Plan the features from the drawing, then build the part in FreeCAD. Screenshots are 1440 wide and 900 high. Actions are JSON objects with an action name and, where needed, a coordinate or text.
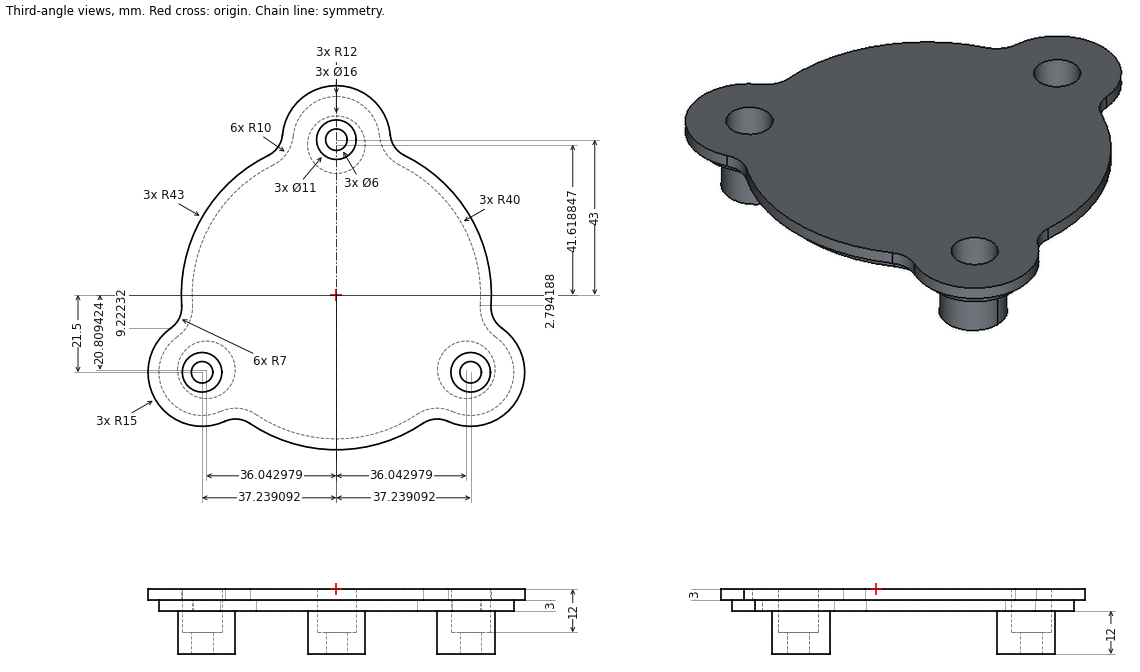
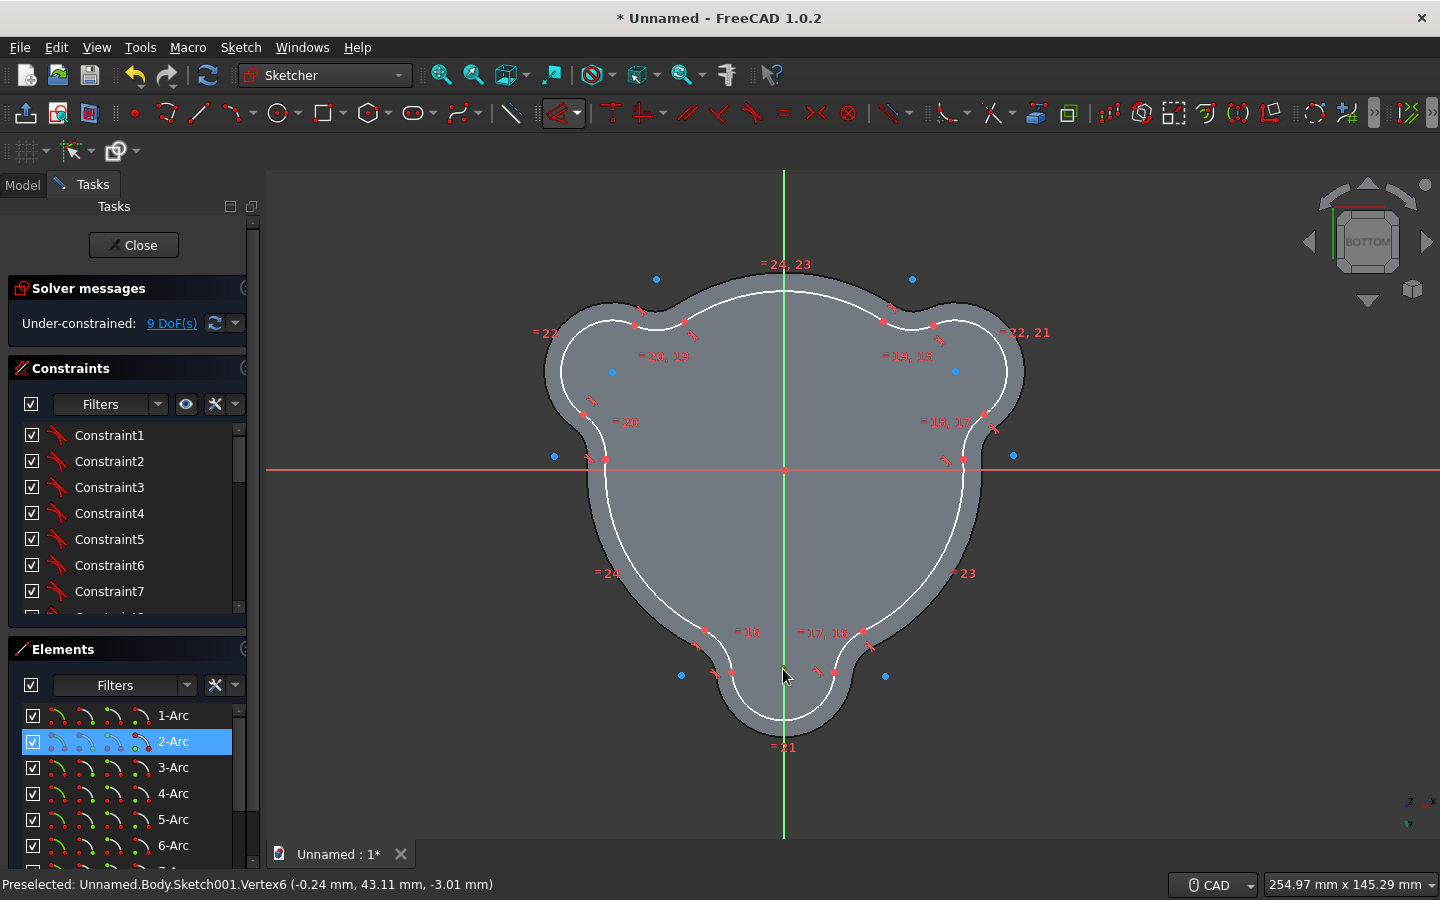
{"action": "left_click", "coordinate": [784, 767]}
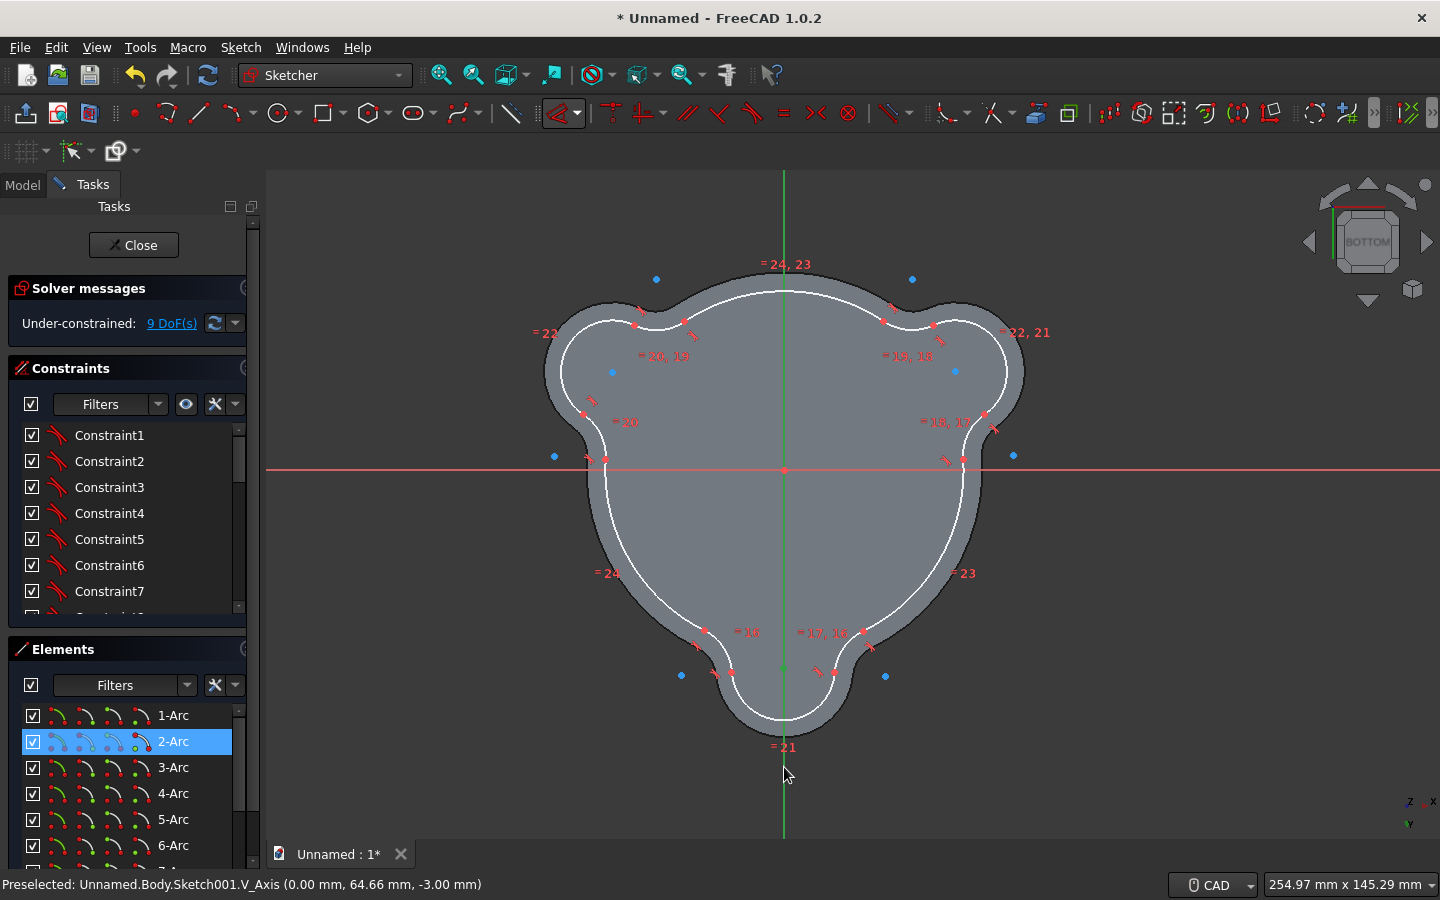
{"action": "left_click", "coordinate": [612, 114]}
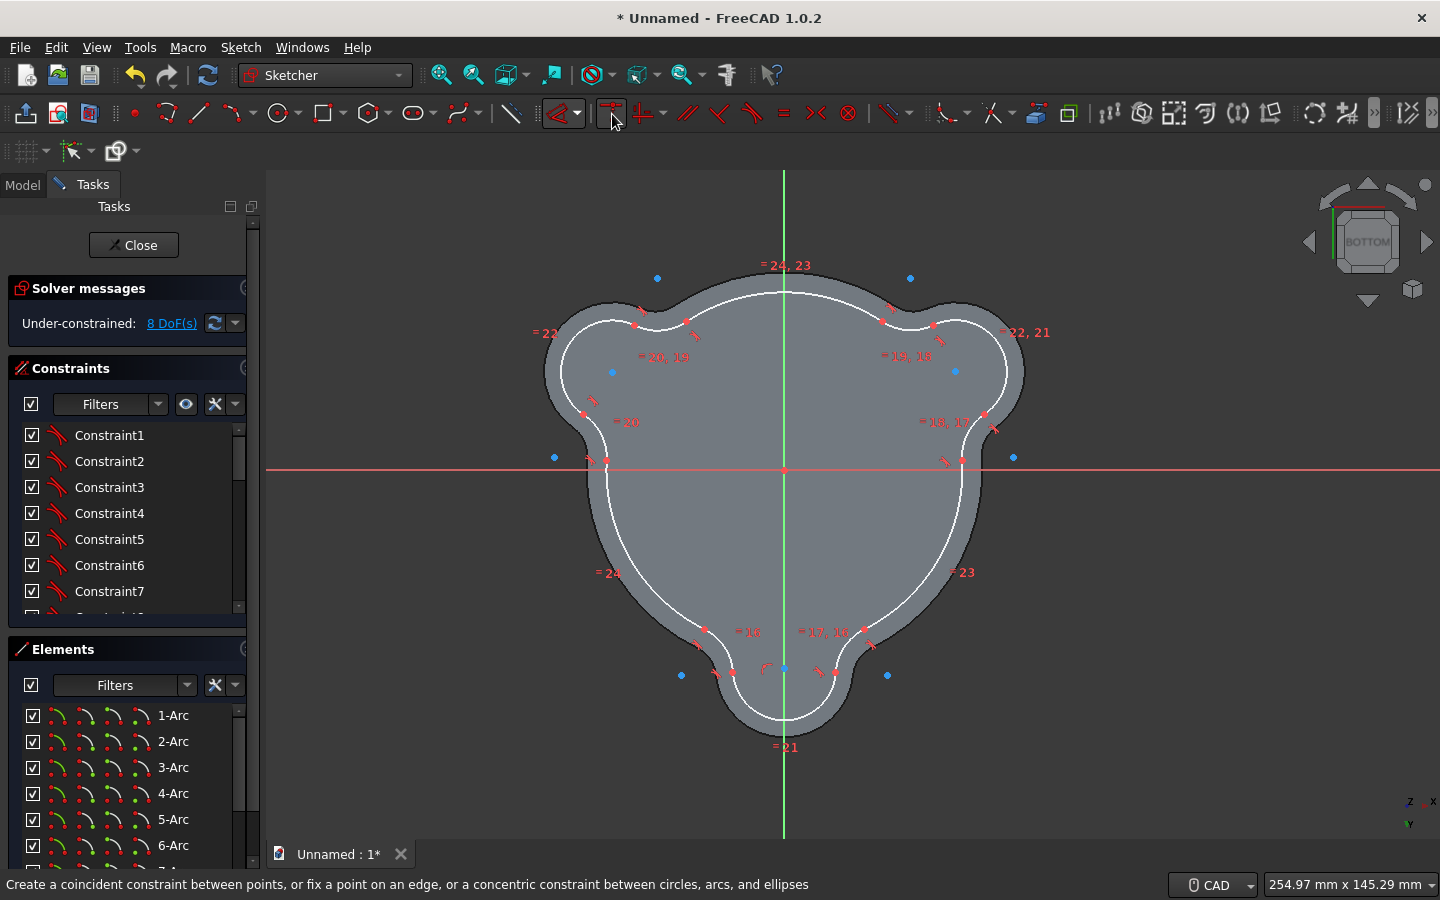
{"action": "left_click", "coordinate": [955, 372]}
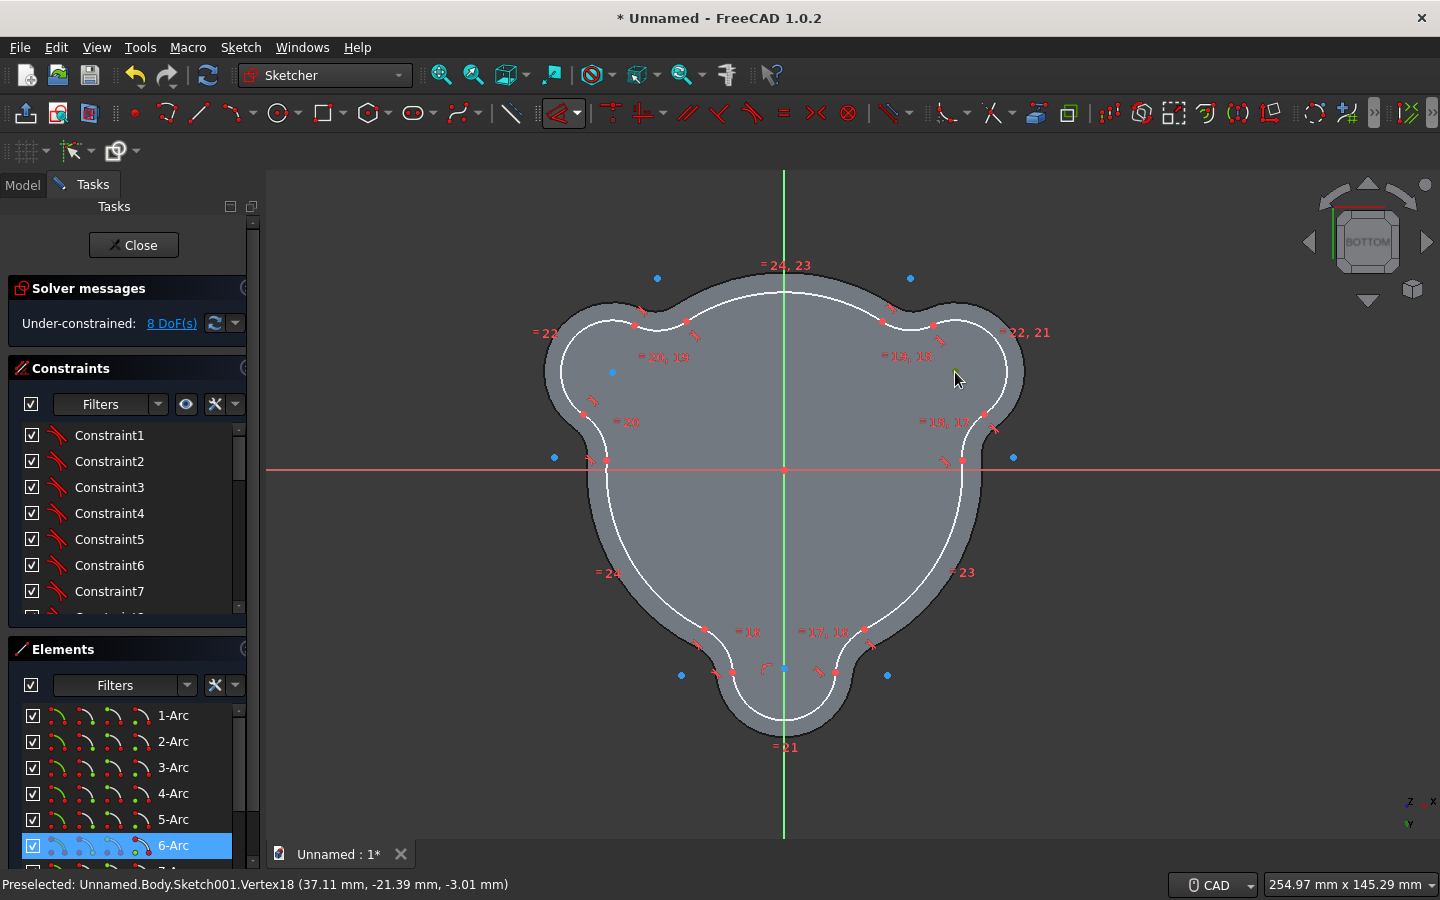
{"action": "left_click", "coordinate": [613, 372]}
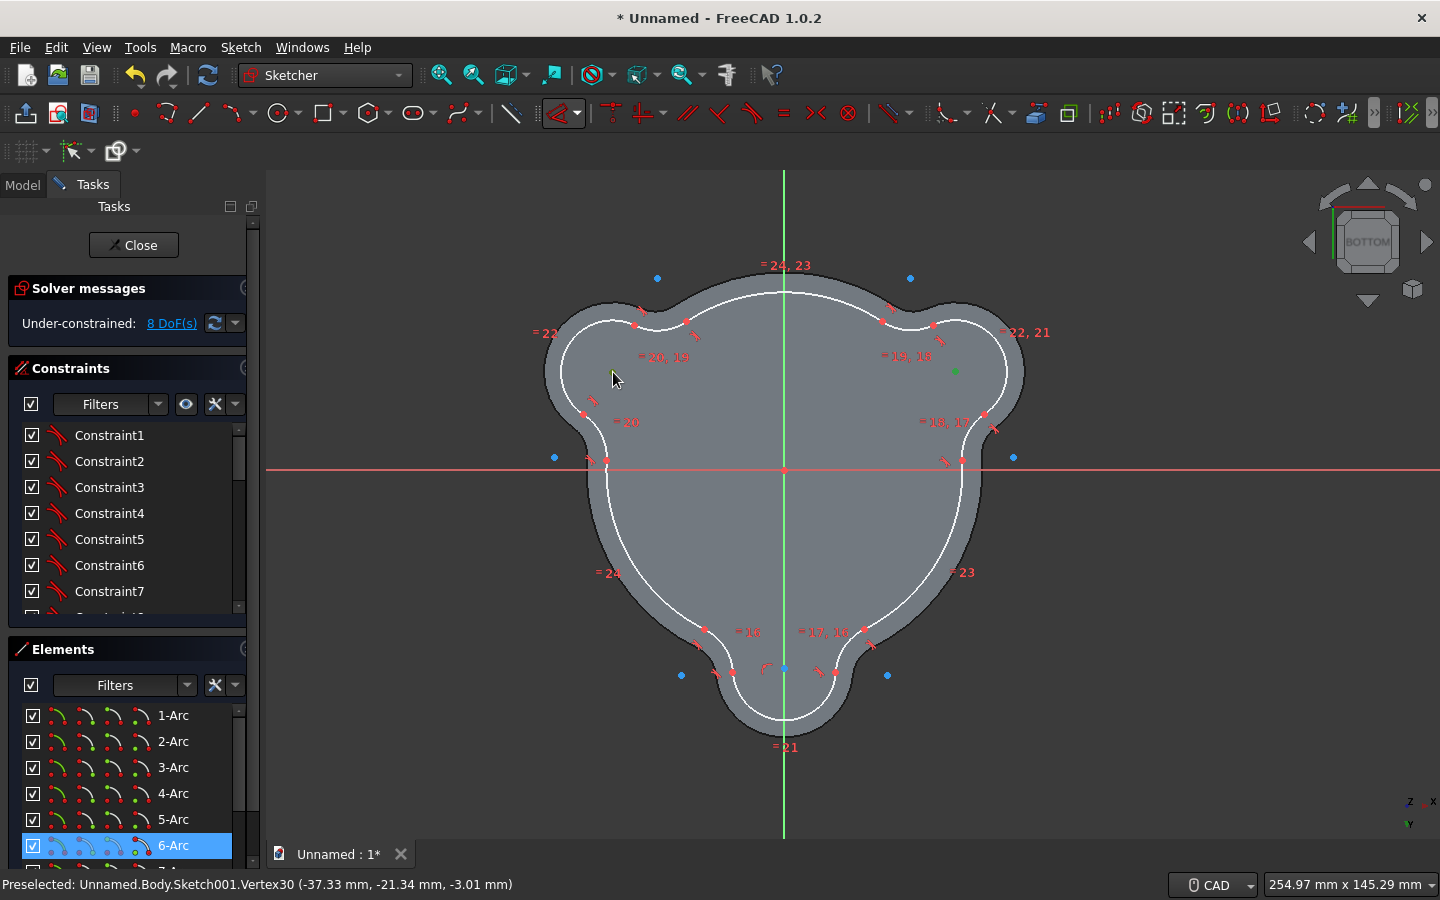
{"action": "left_click", "coordinate": [784, 767]}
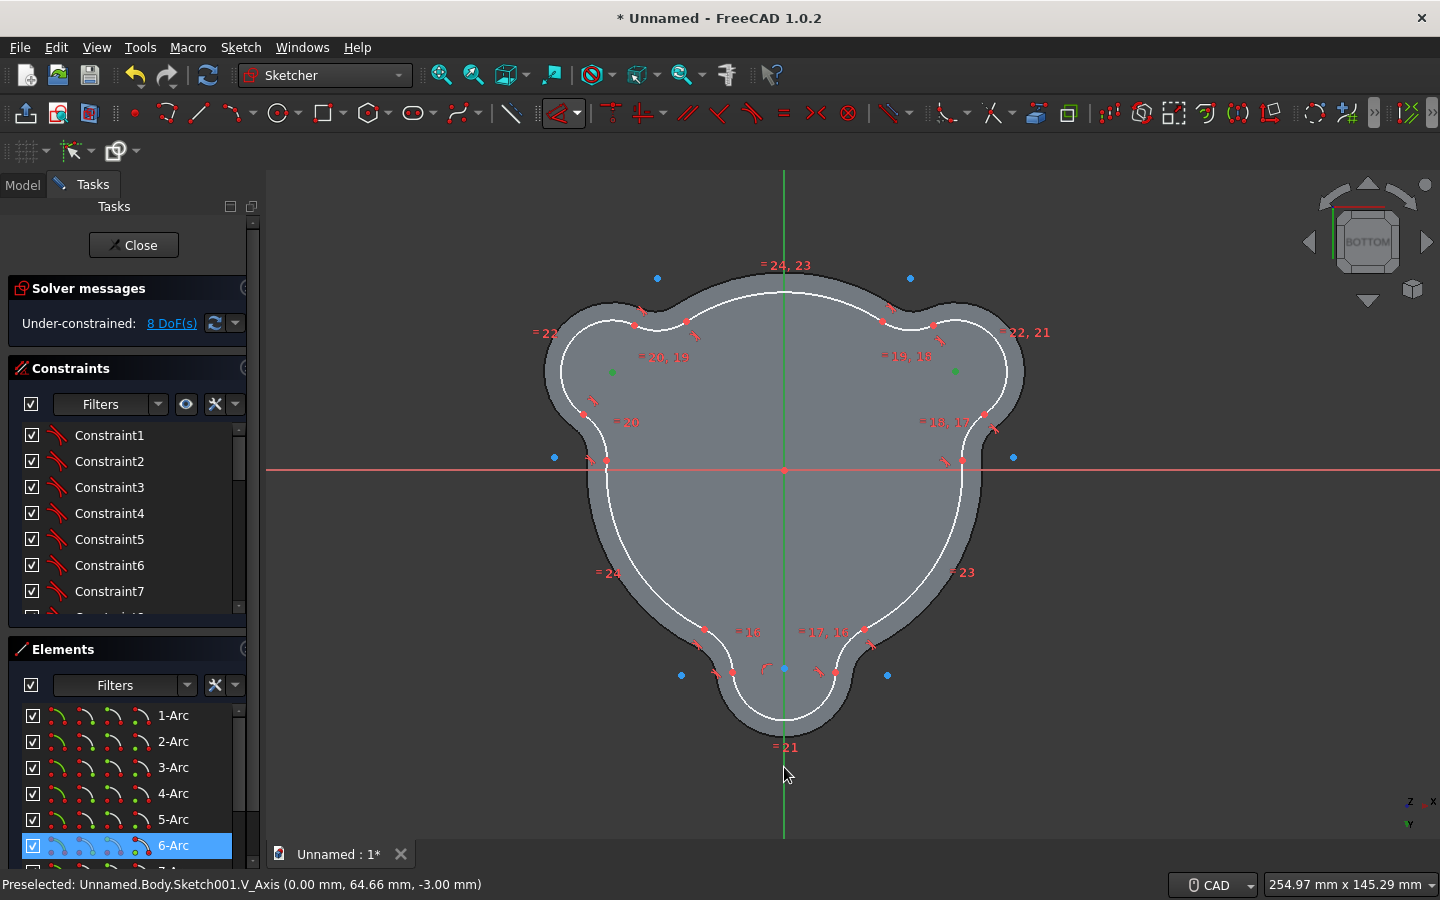
{"action": "left_click", "coordinate": [816, 114]}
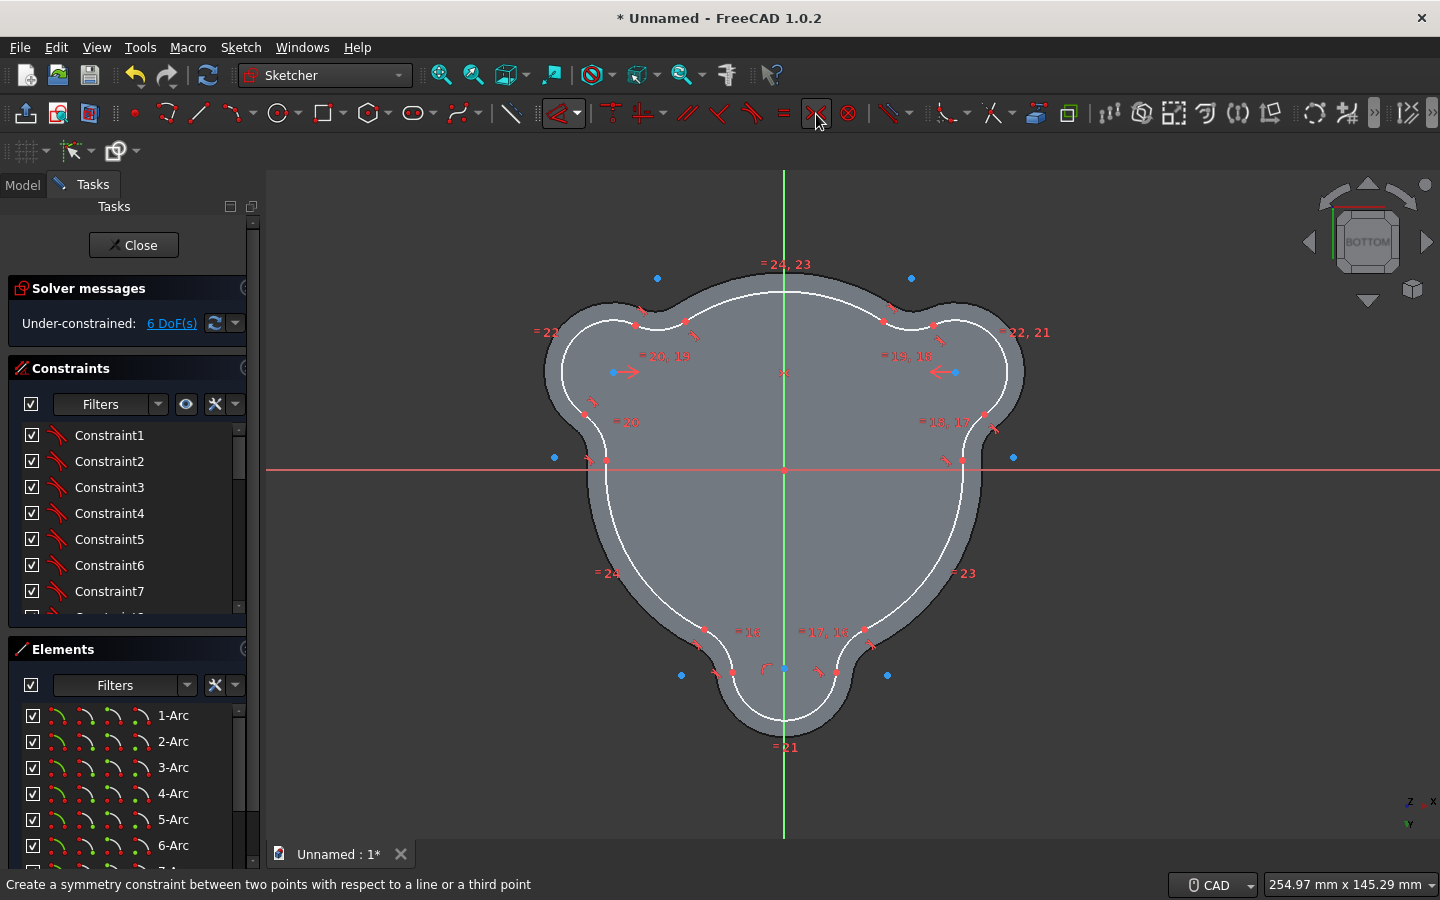
{"action": "left_click", "coordinate": [729, 657]}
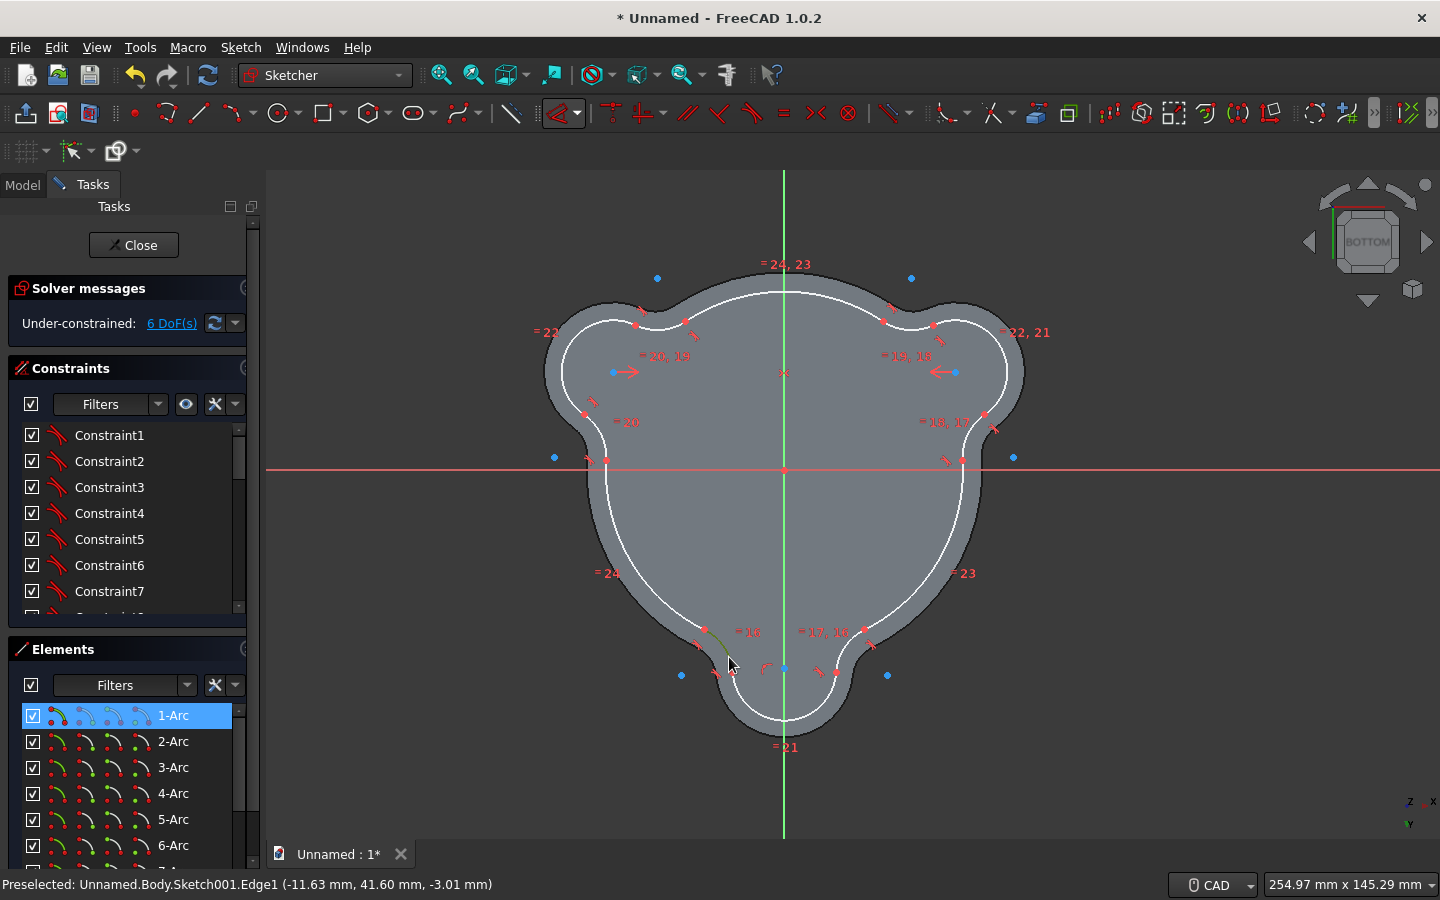
{"action": "left_click", "coordinate": [580, 114]}